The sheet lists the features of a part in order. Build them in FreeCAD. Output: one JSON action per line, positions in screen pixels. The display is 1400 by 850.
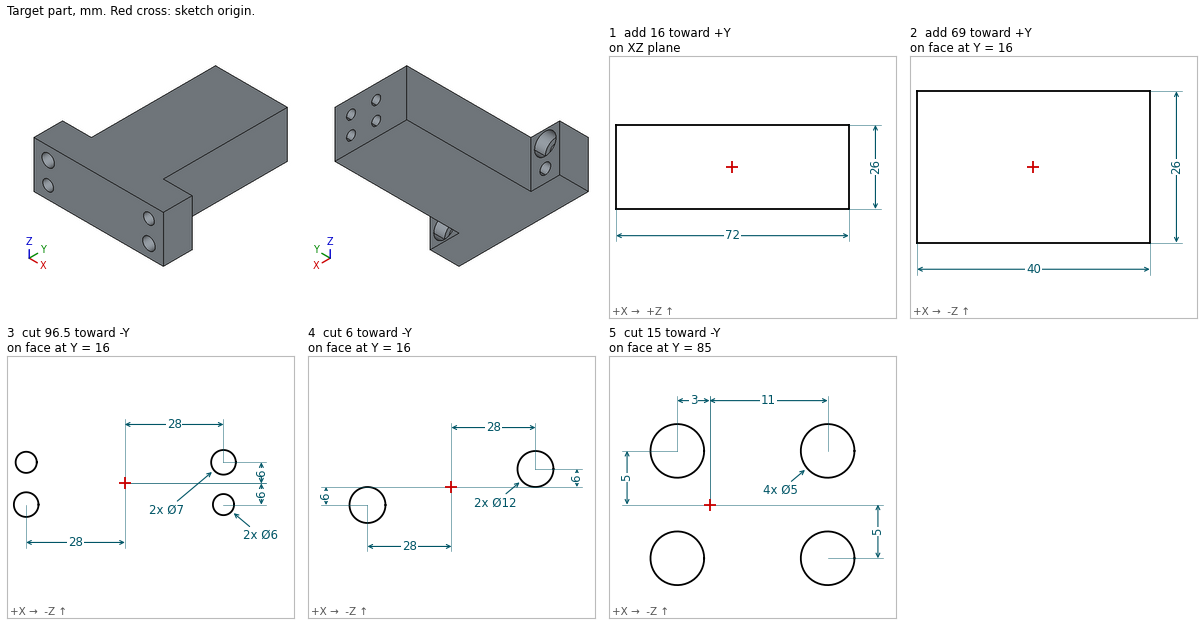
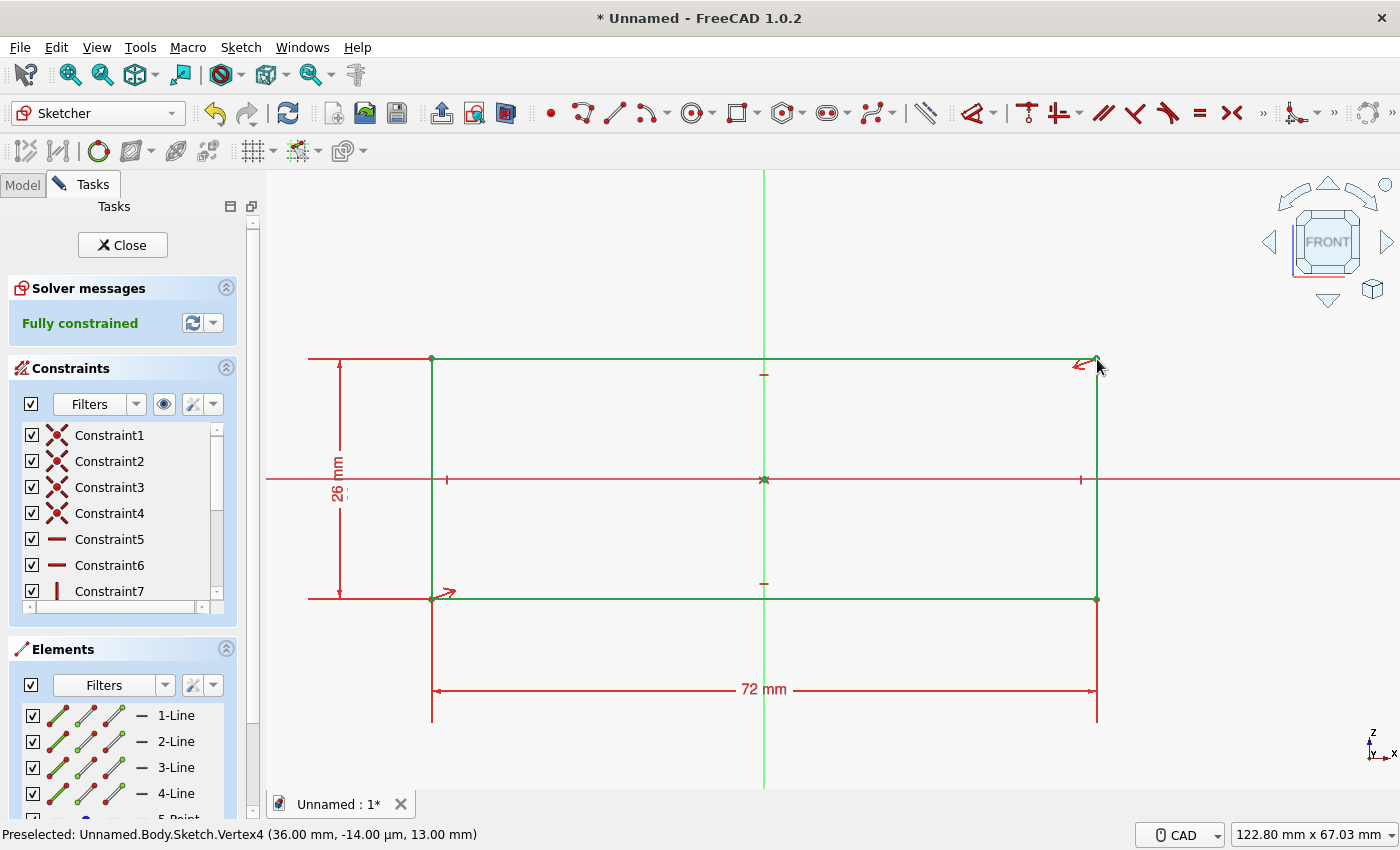
{"action": "left_click", "coordinate": [123, 245]}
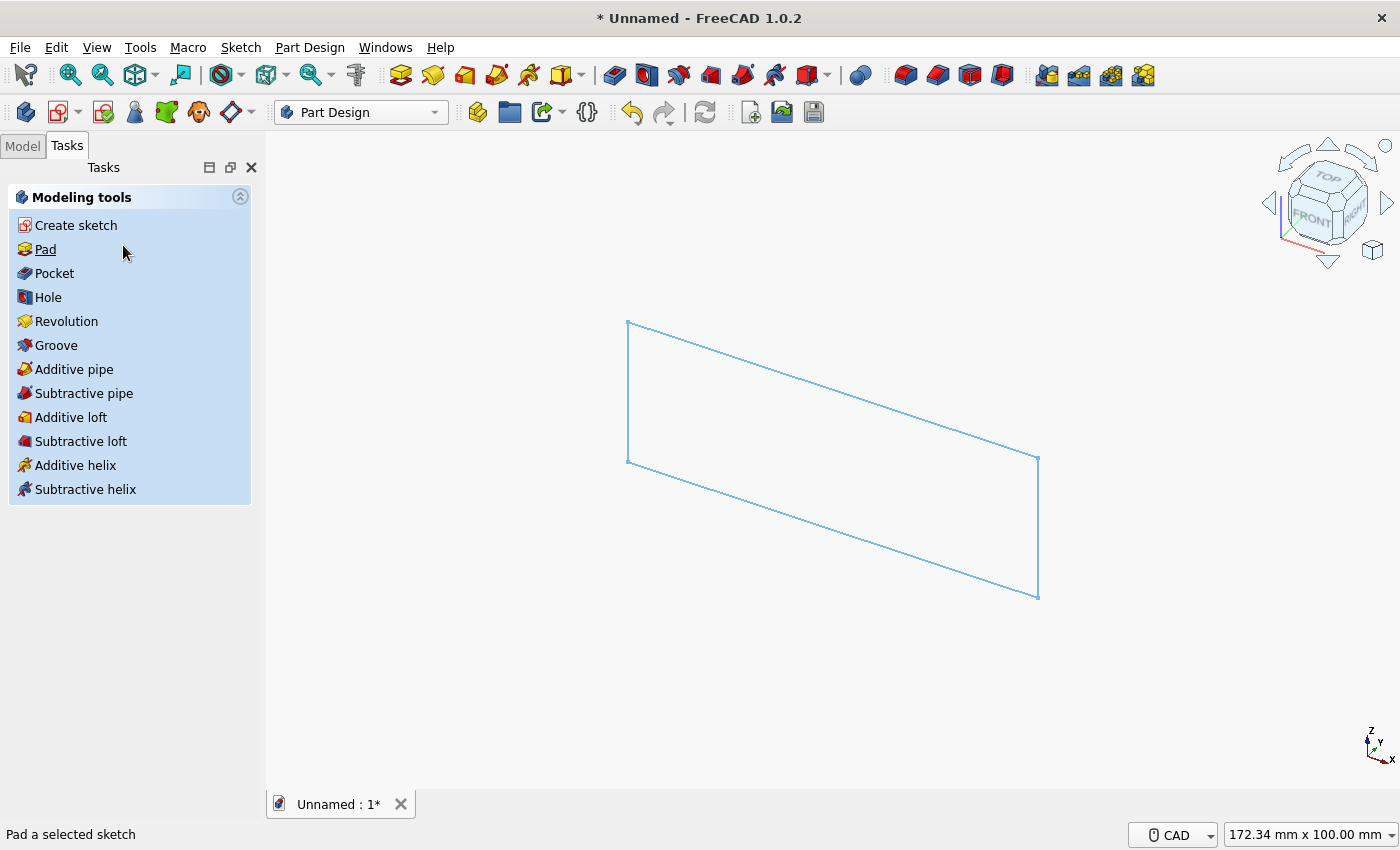
{"action": "left_click", "coordinate": [402, 76]}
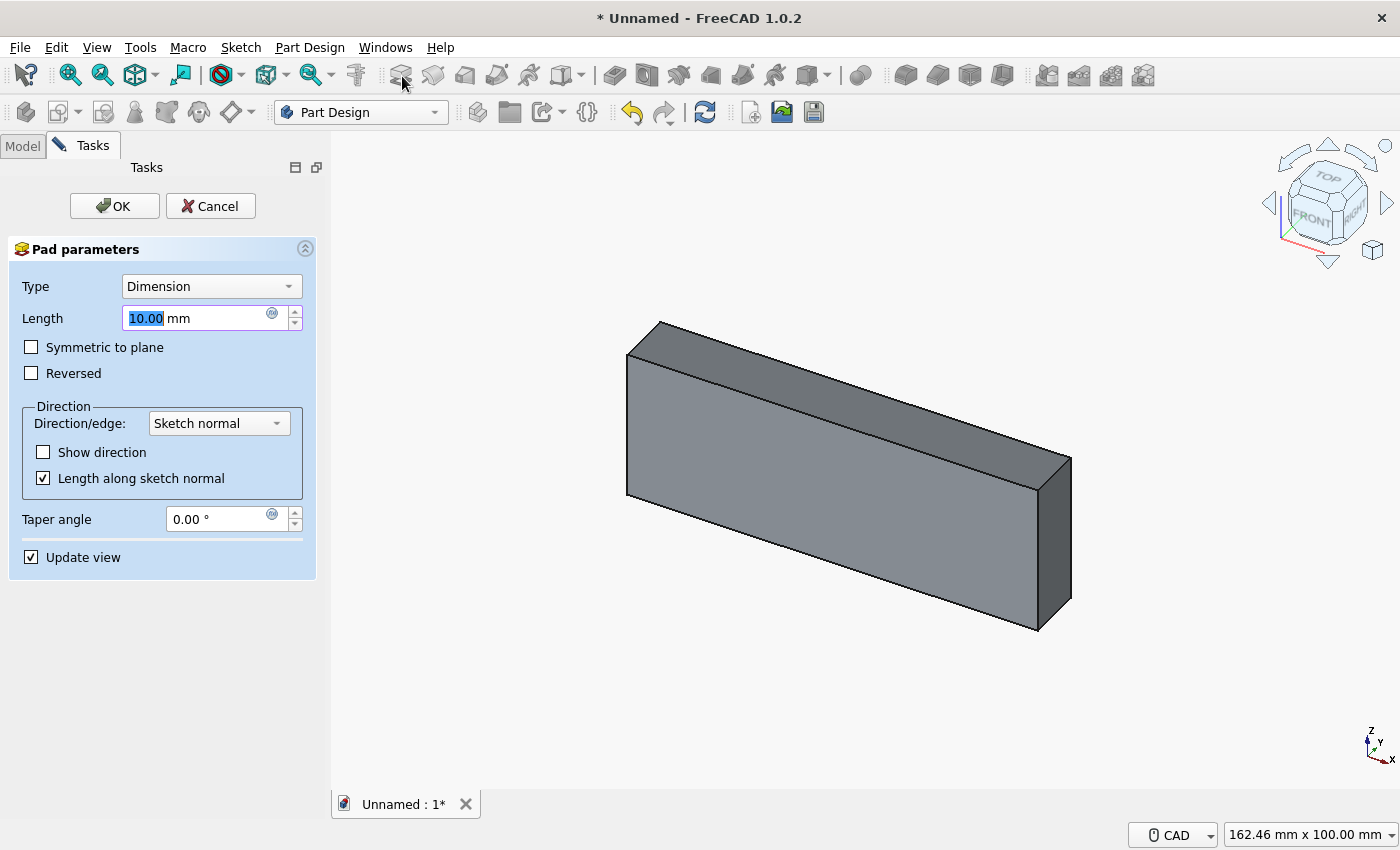
{"action": "type", "text": "16"}
{"action": "key", "text": "Tab"}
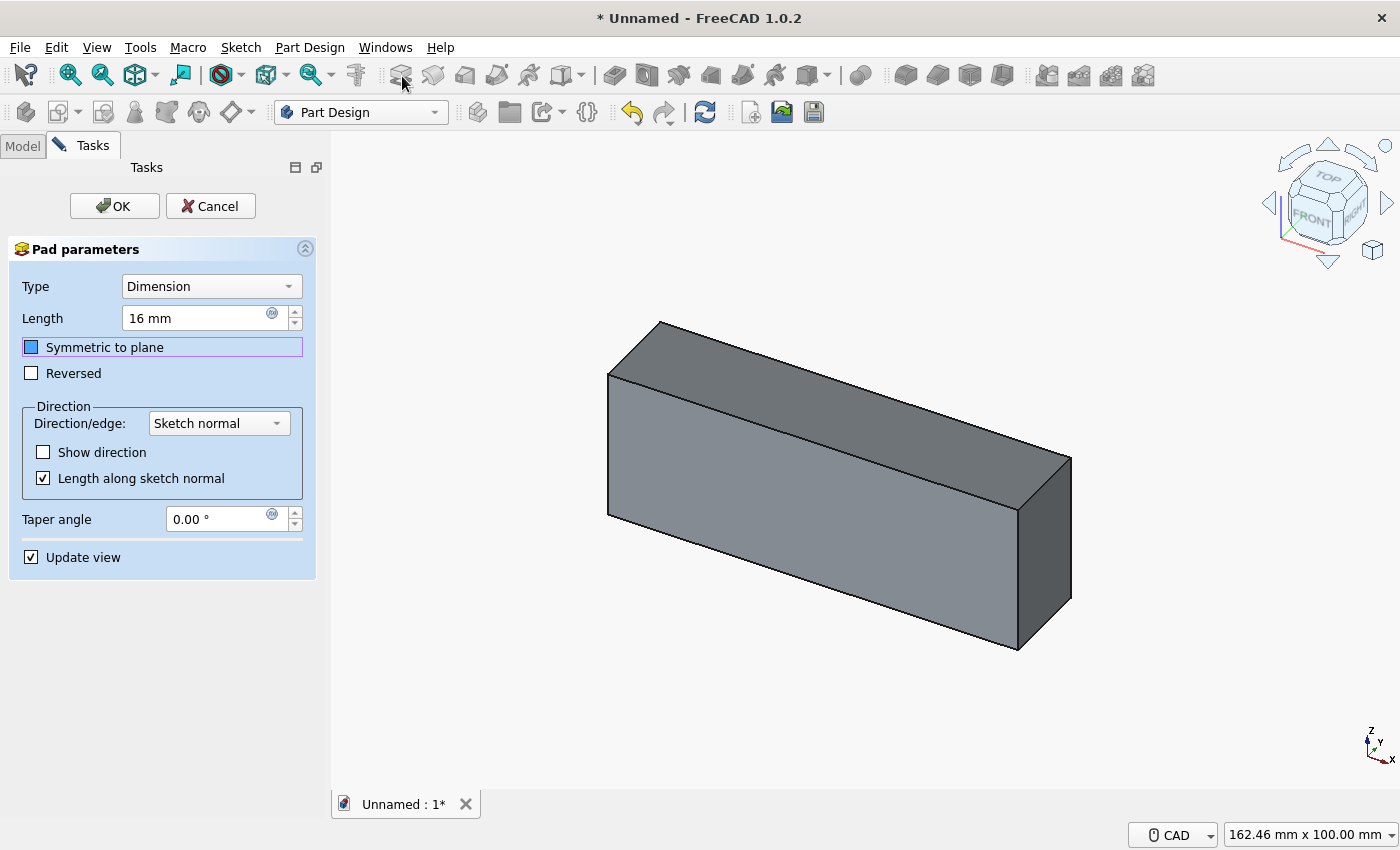
{"action": "left_click", "coordinate": [30, 373]}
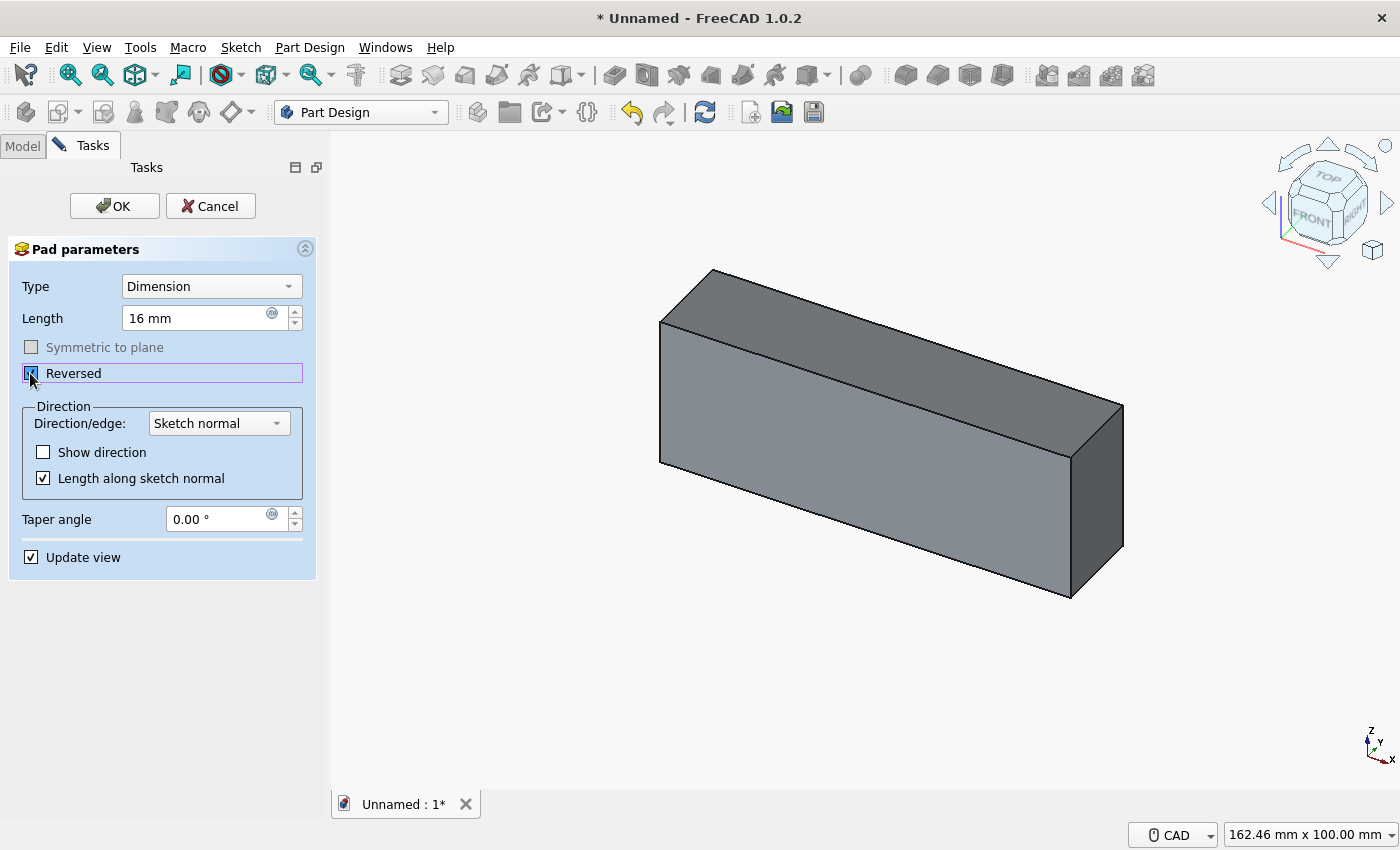
{"action": "left_click", "coordinate": [115, 206]}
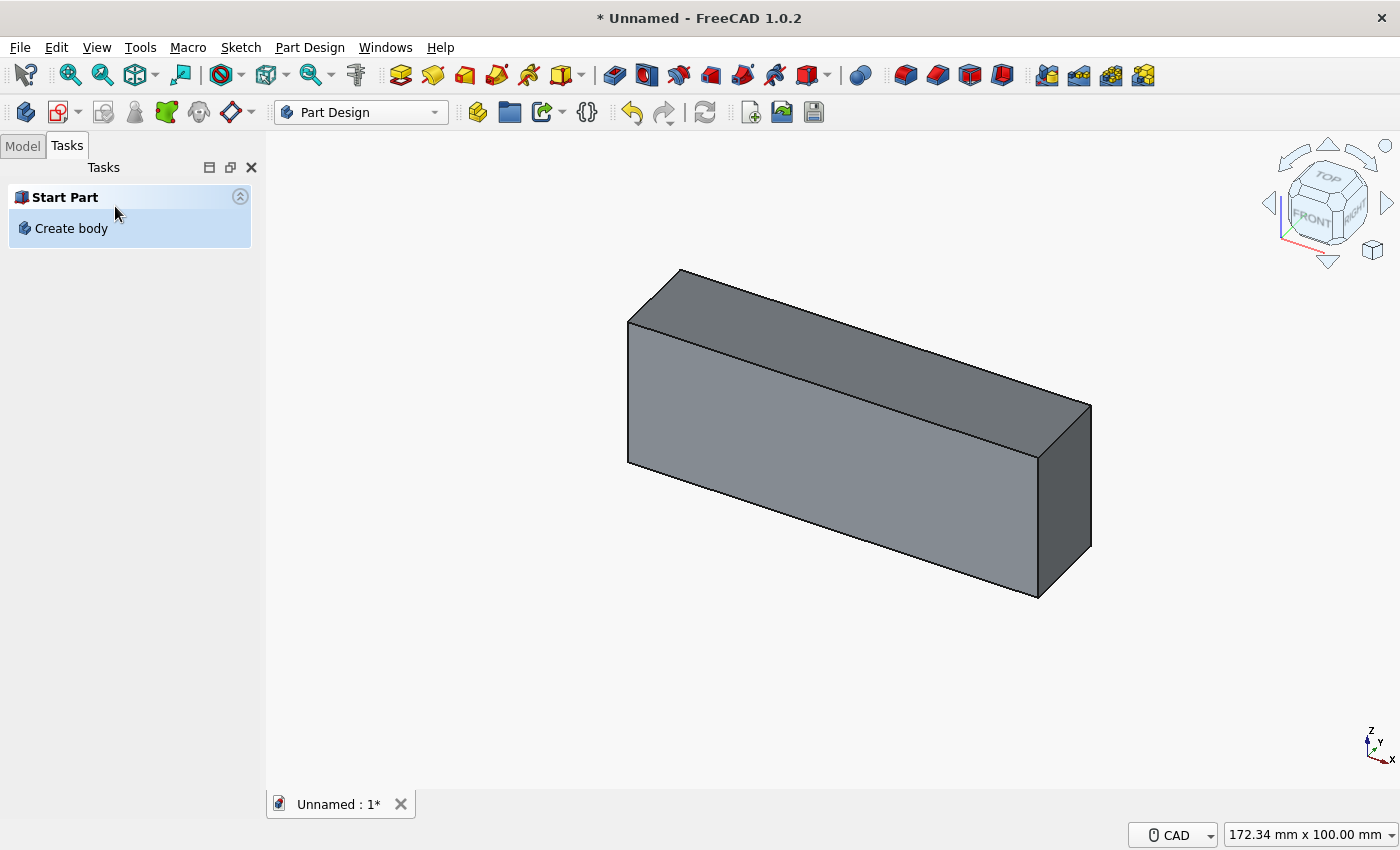
{"action": "key", "text": "4"}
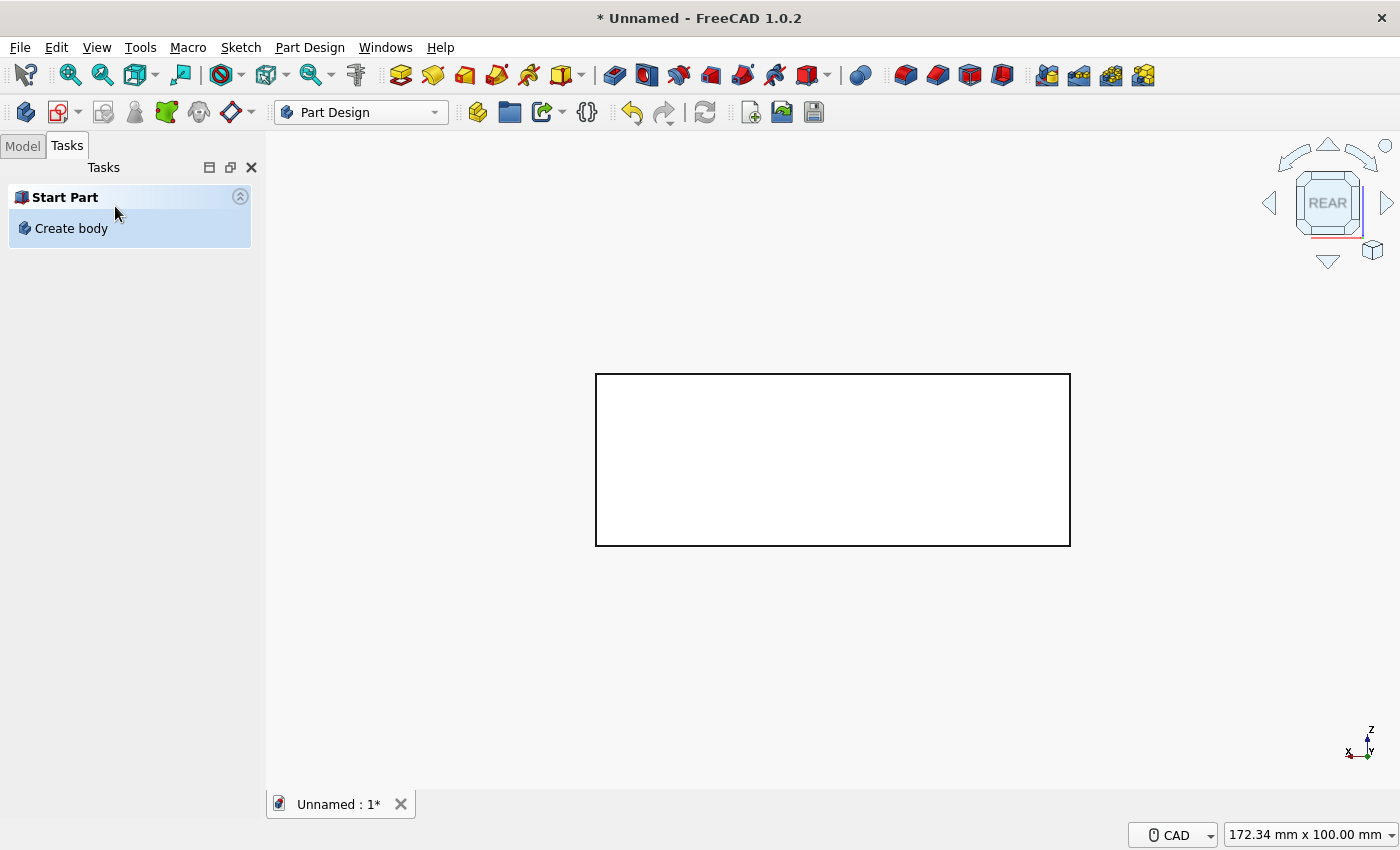
{"action": "key", "text": "v f"}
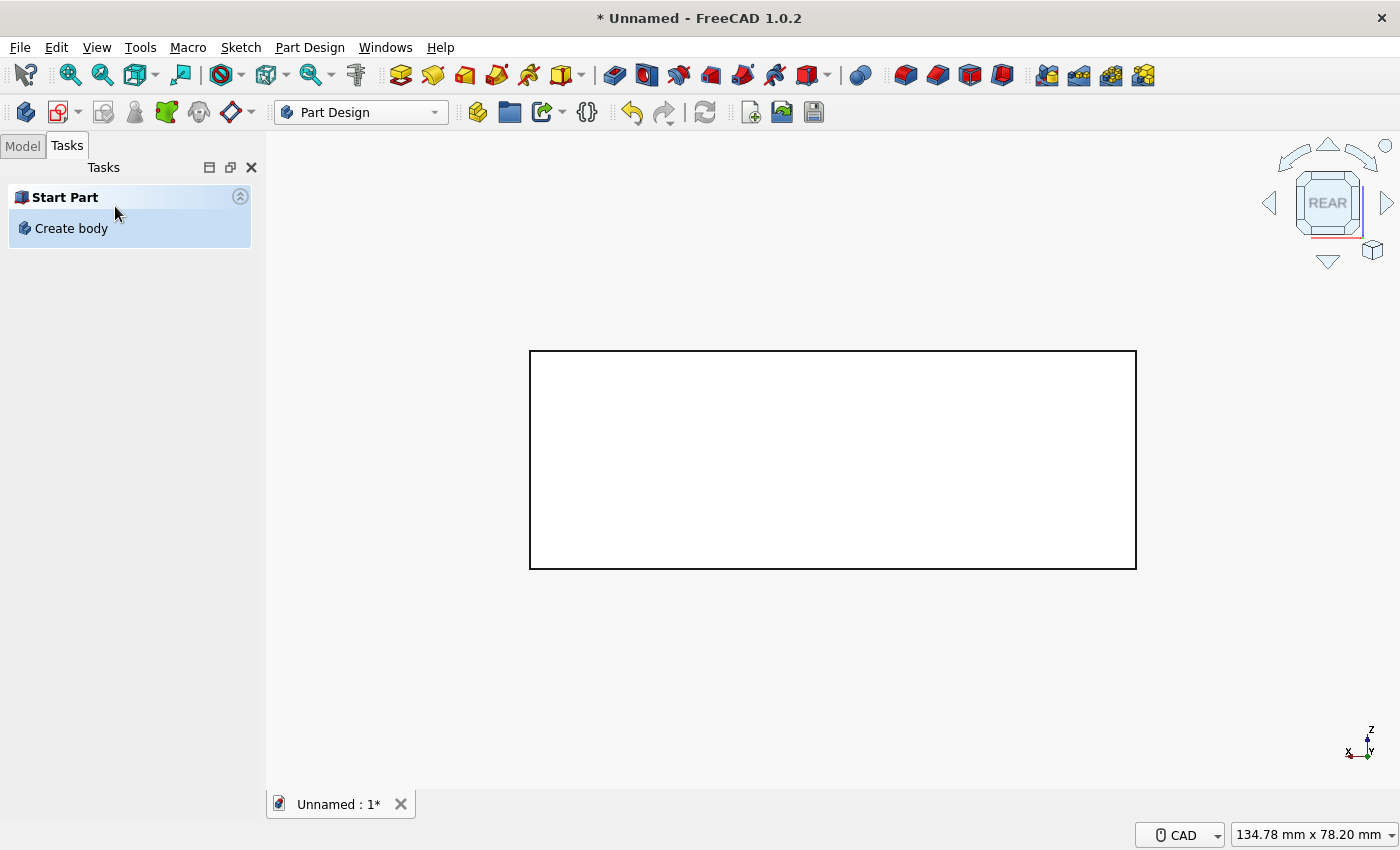
{"action": "left_click", "coordinate": [660, 459]}